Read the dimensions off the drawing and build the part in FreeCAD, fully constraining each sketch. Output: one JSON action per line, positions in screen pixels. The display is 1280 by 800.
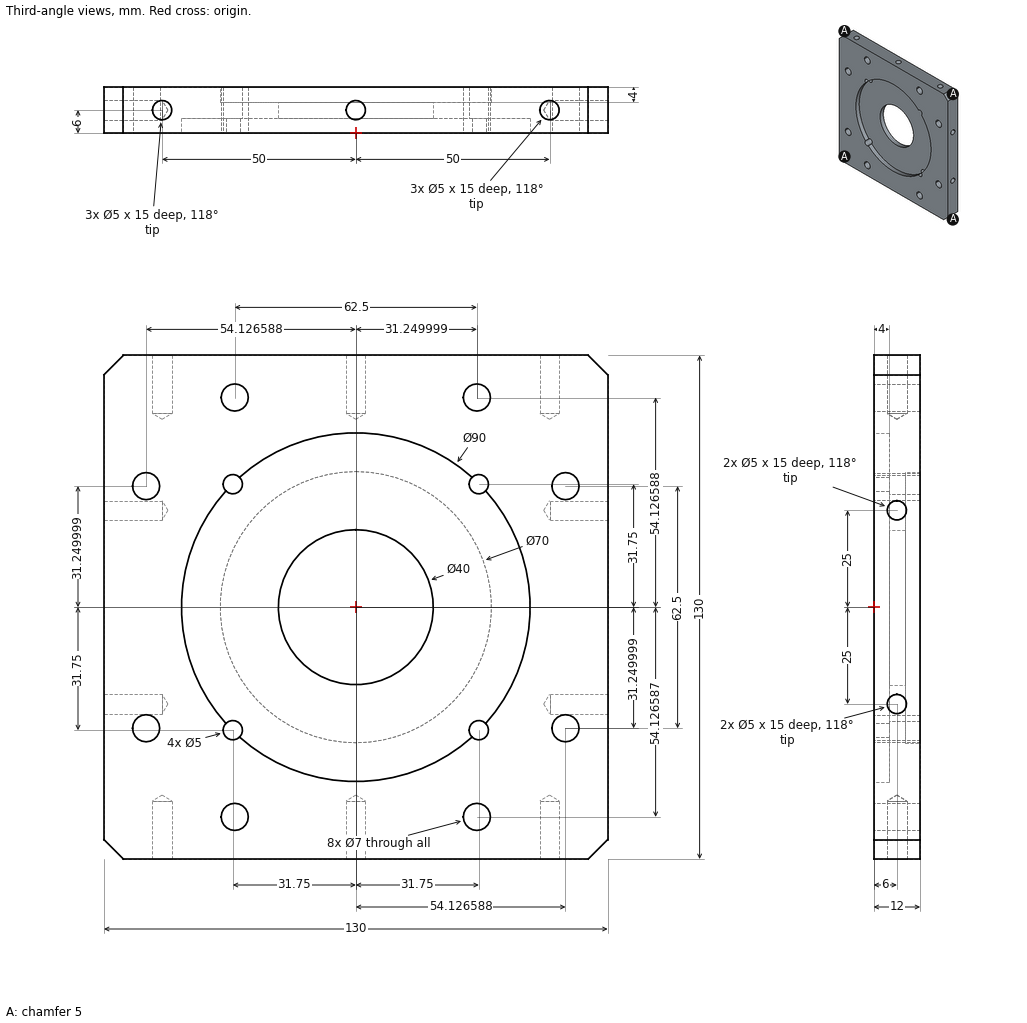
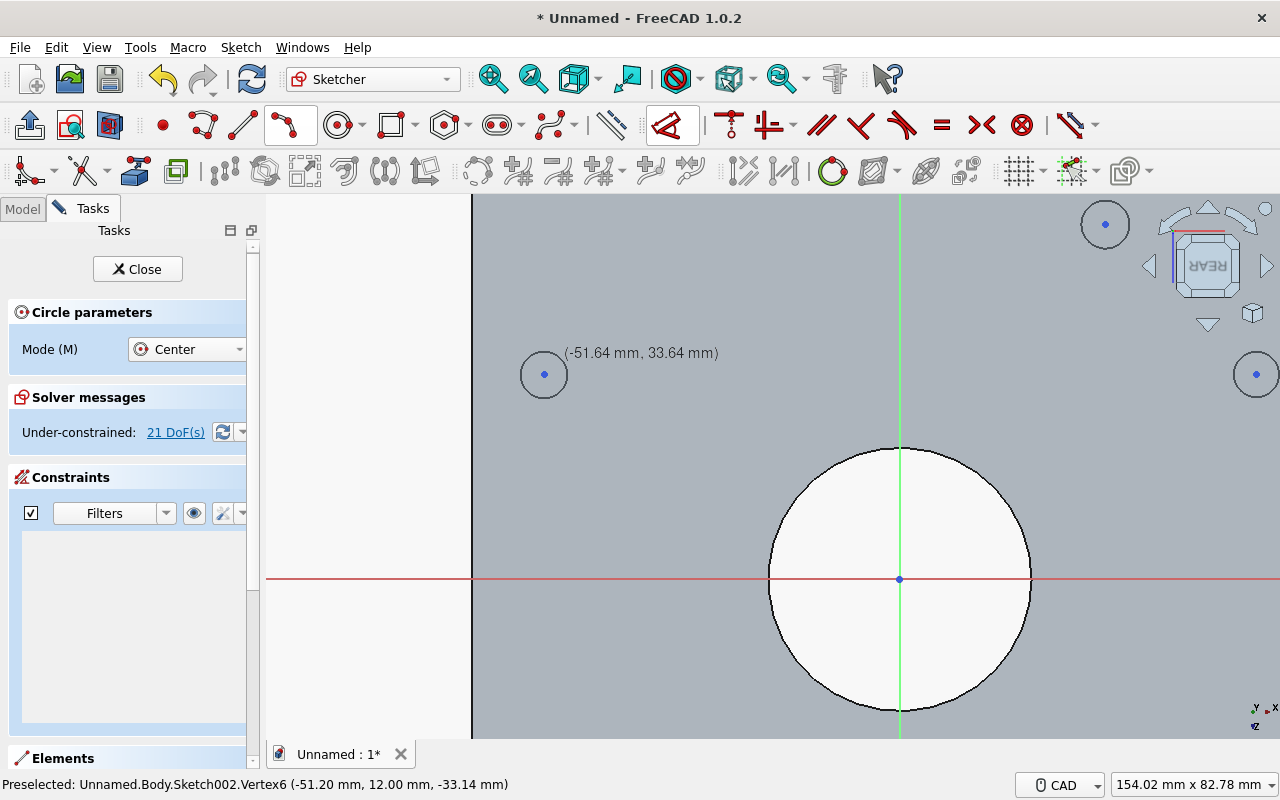
{"action": "left_click", "coordinate": [694, 223]}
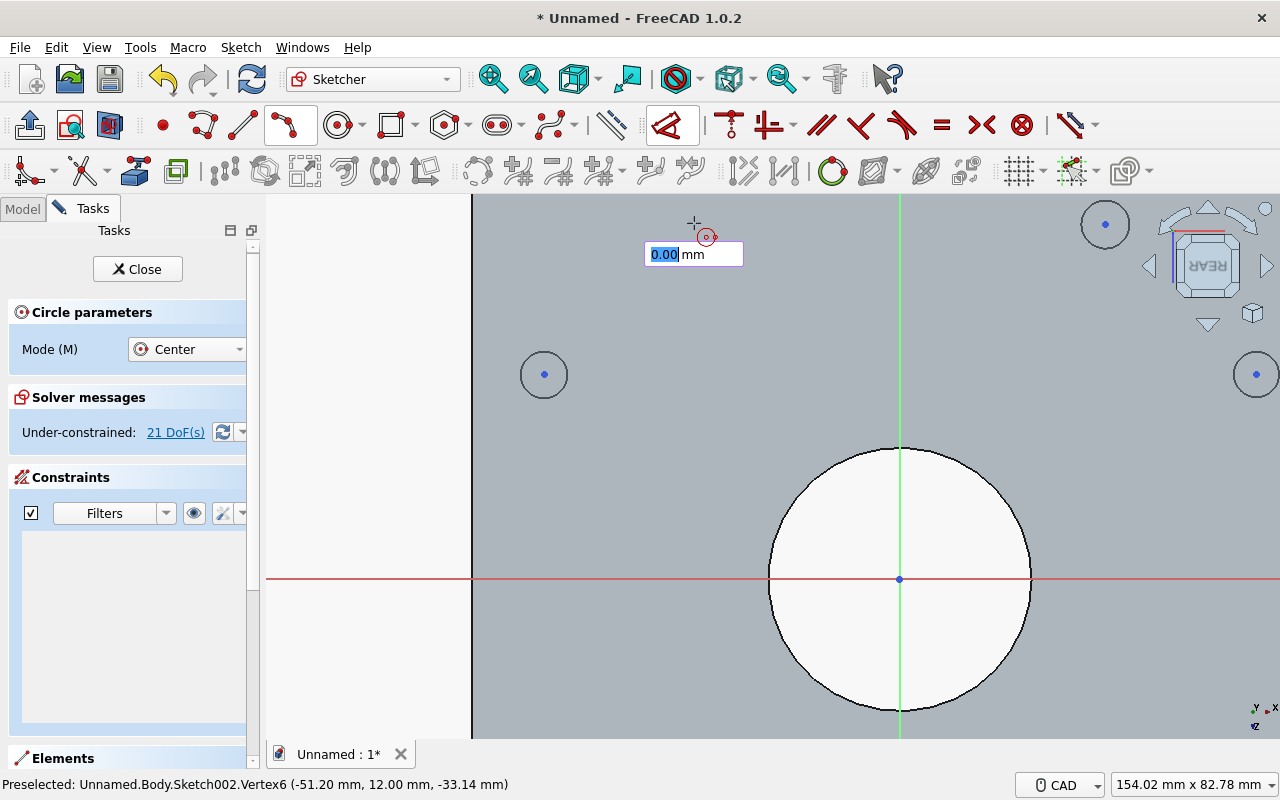
{"action": "scroll", "coordinate": [545, 374], "scroll_direction": "down", "scroll_amount": 4}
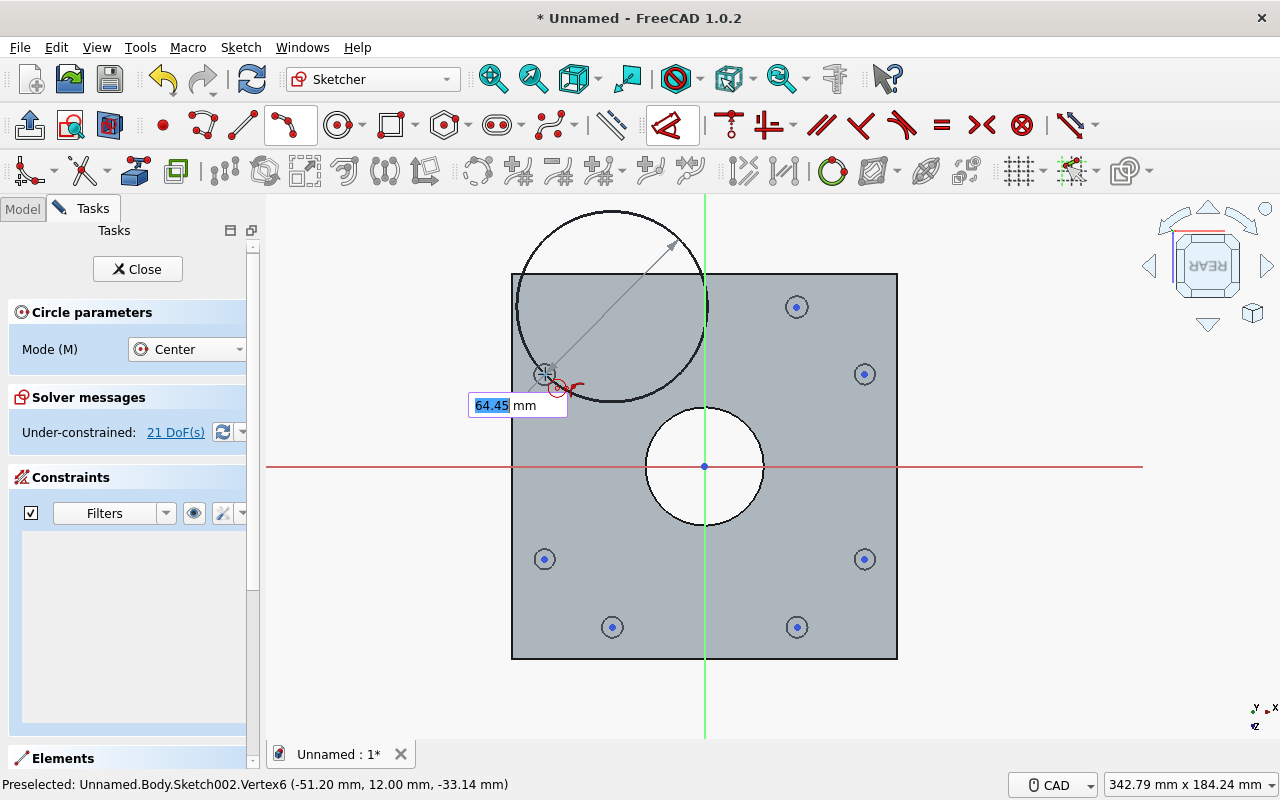
{"action": "scroll", "coordinate": [620, 299], "scroll_direction": "up", "scroll_amount": 3}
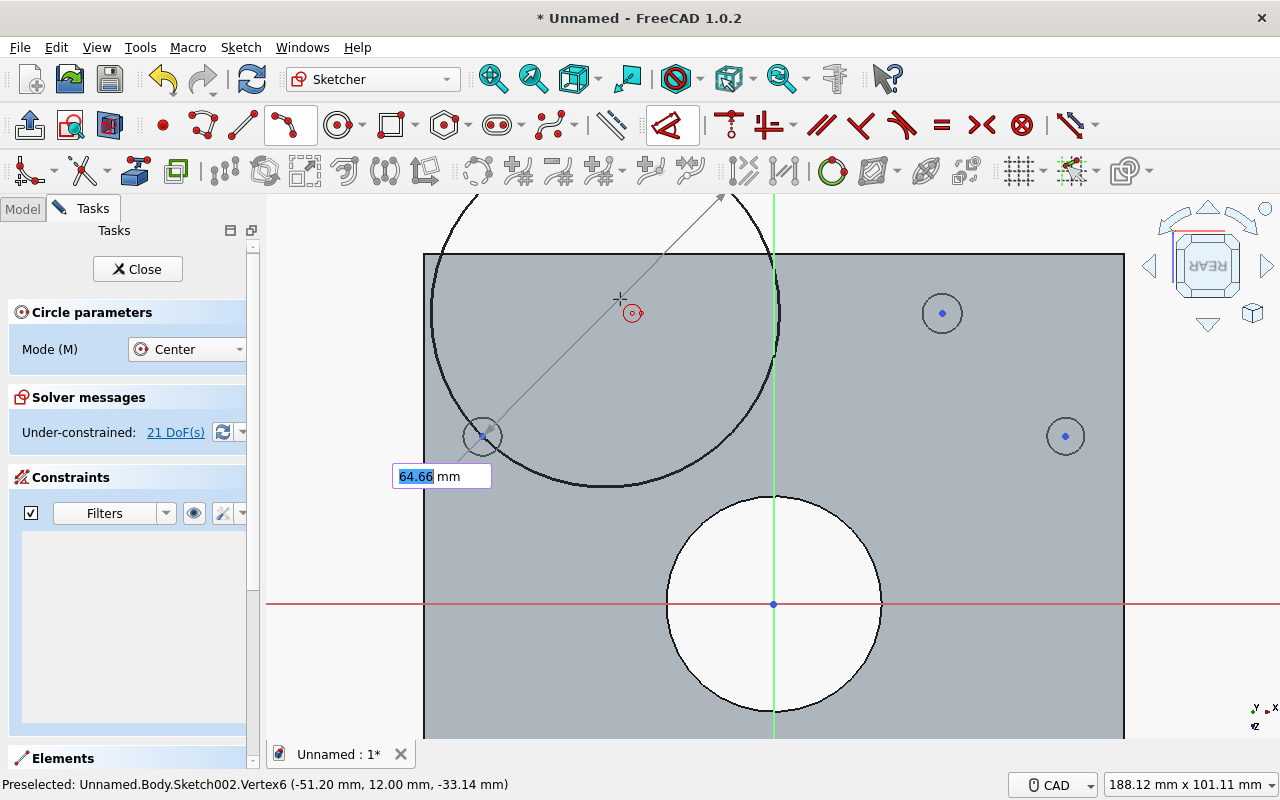
{"action": "left_click", "coordinate": [619, 299]}
{"action": "key", "text": "Escape"}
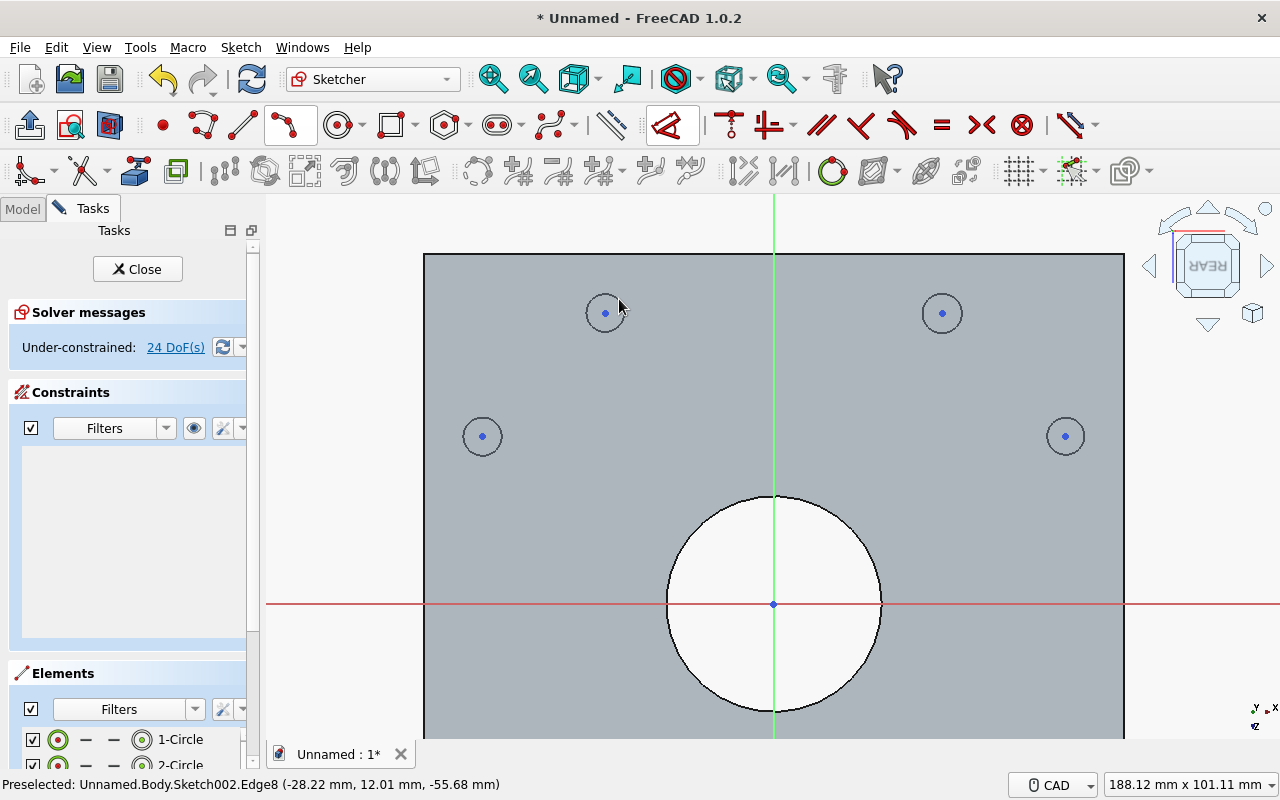
{"action": "left_click", "coordinate": [956, 299]}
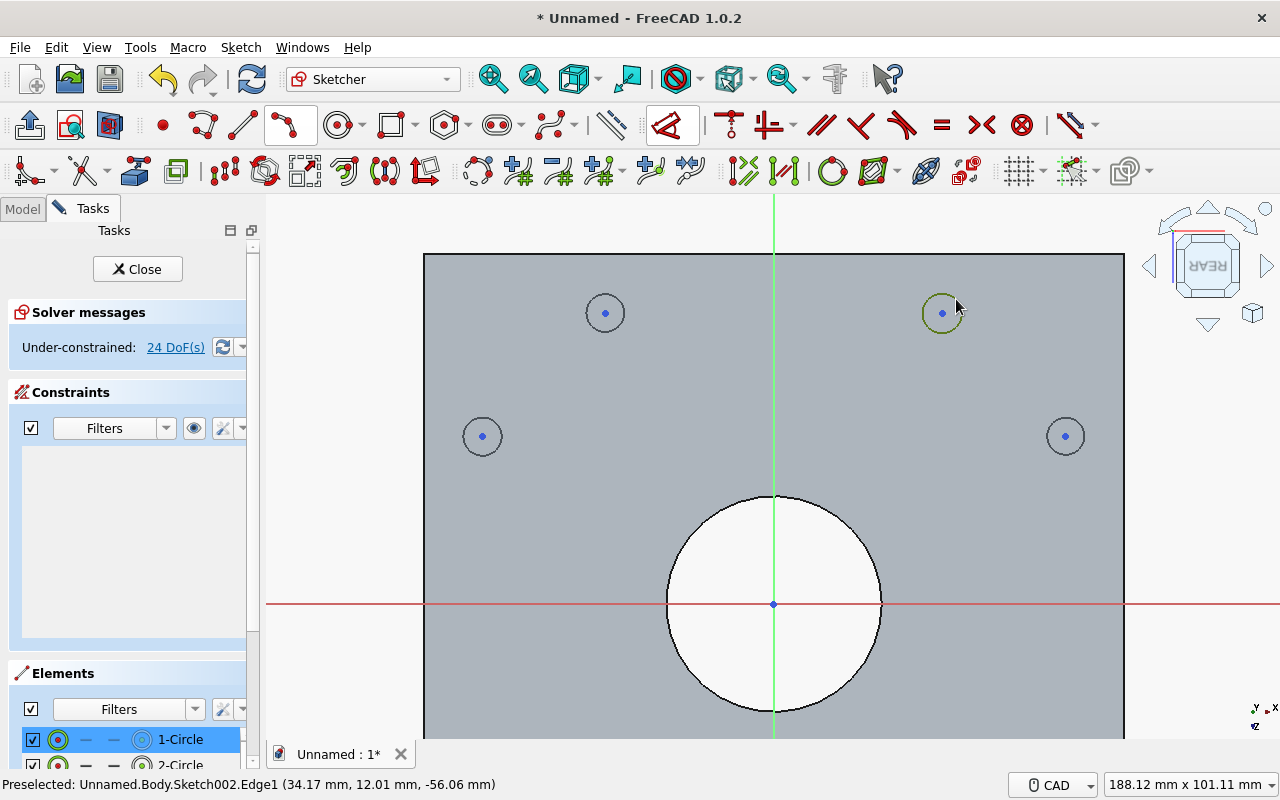
{"action": "left_click", "coordinate": [1079, 423]}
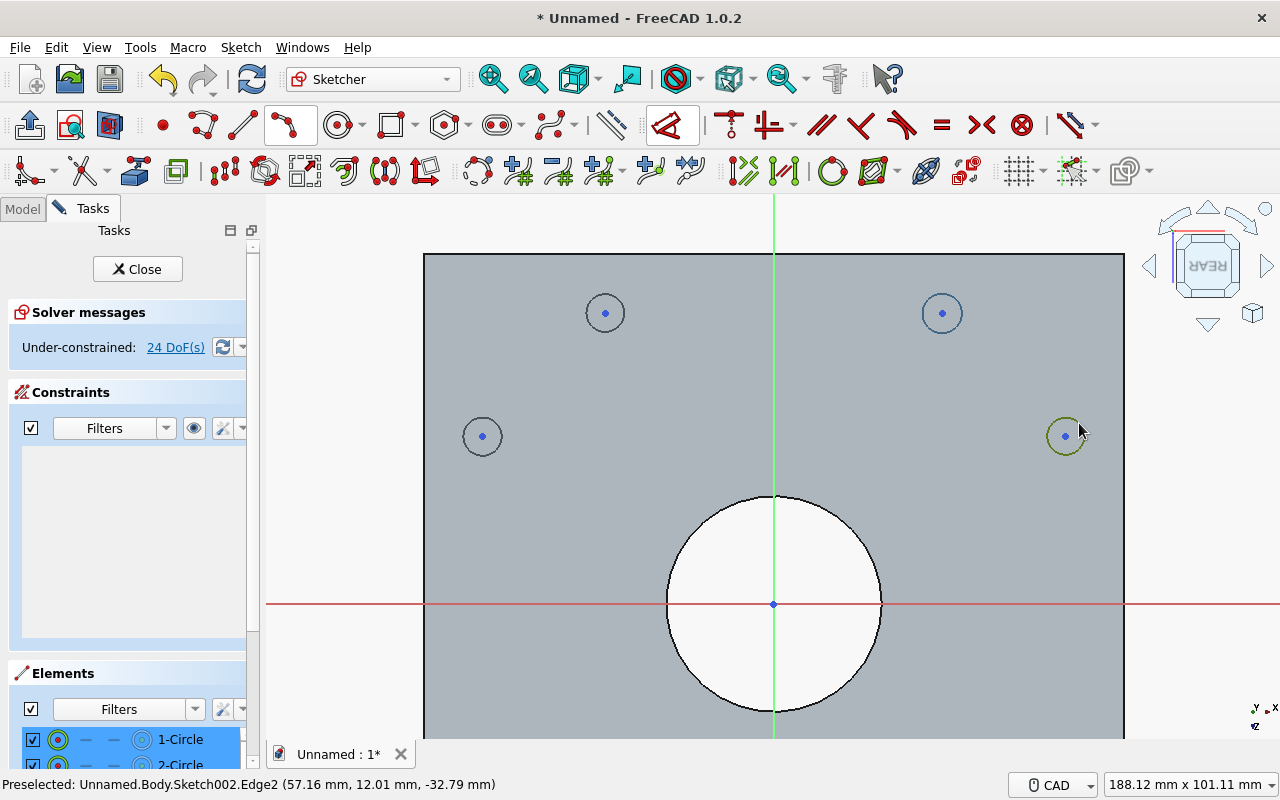
{"action": "scroll", "coordinate": [620, 299], "scroll_direction": "down", "scroll_amount": 3}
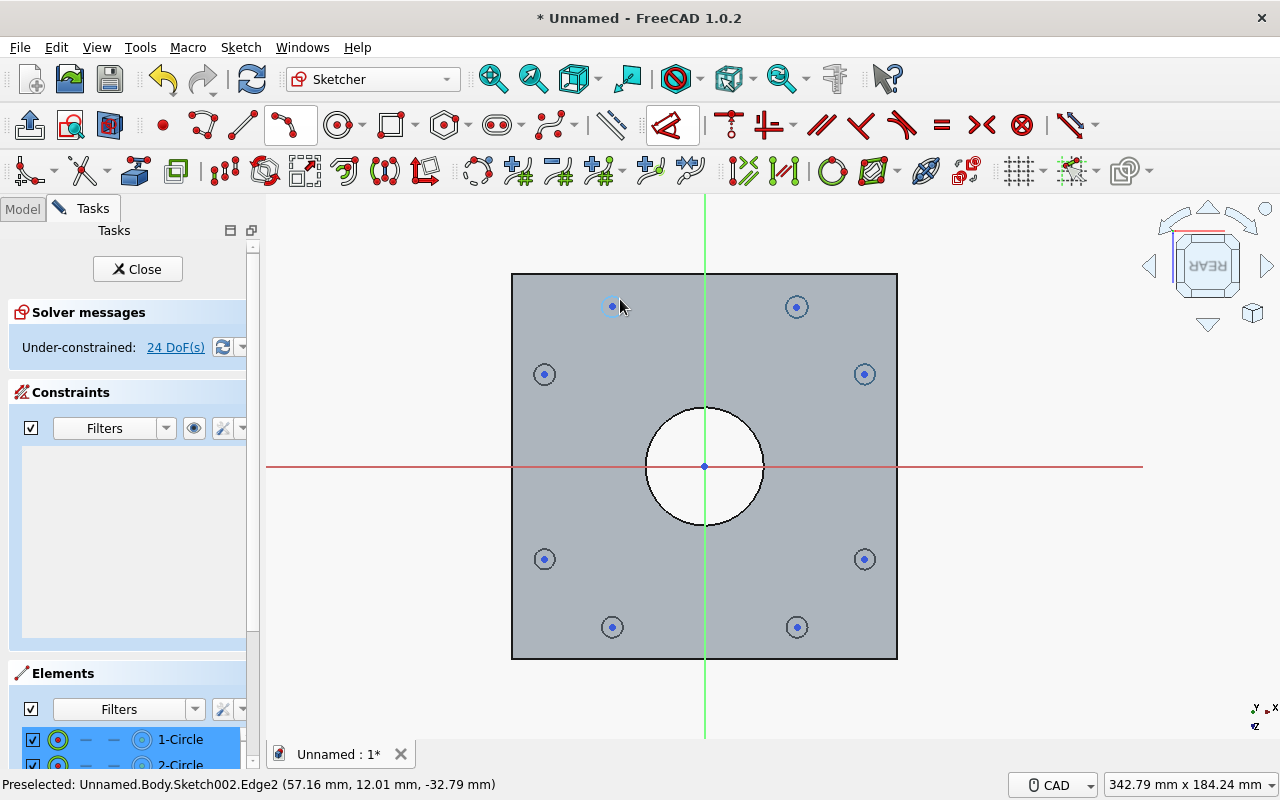
{"action": "scroll", "coordinate": [872, 552], "scroll_direction": "up", "scroll_amount": 2}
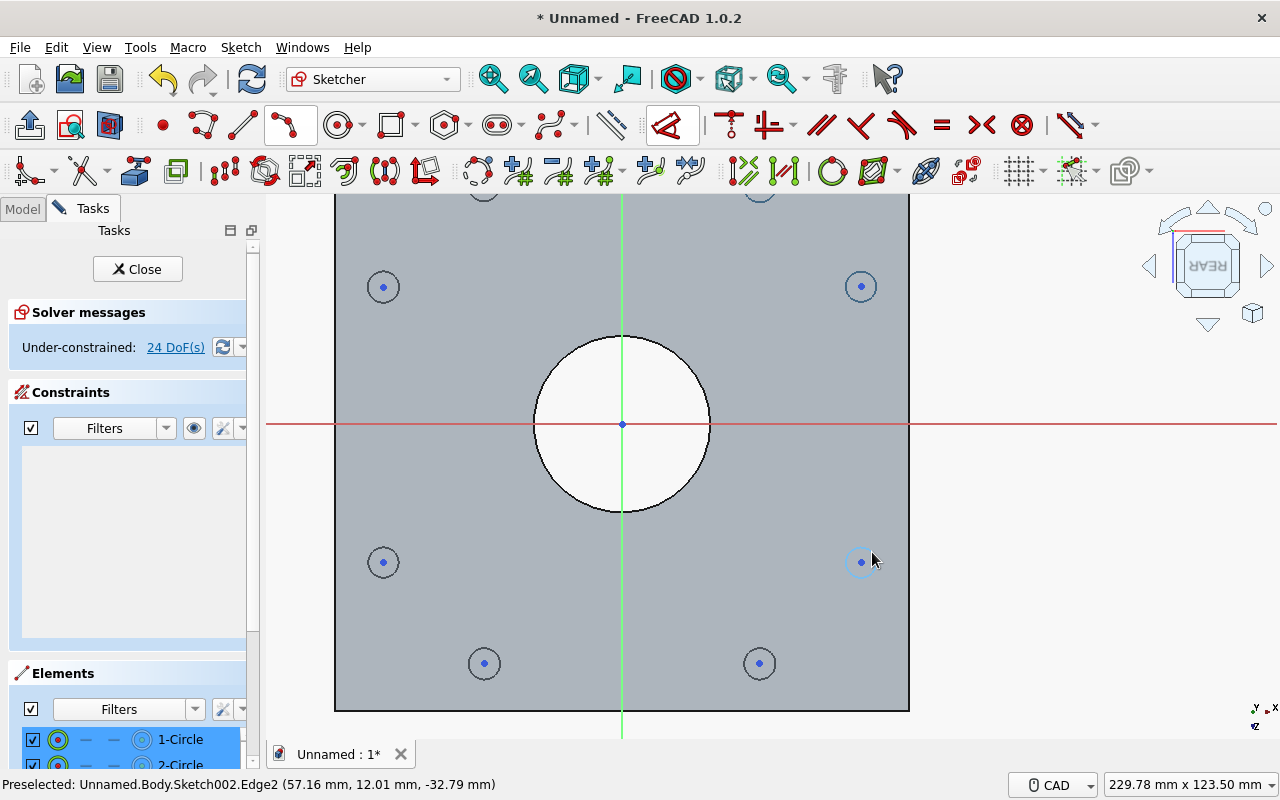
{"action": "left_click", "coordinate": [872, 552]}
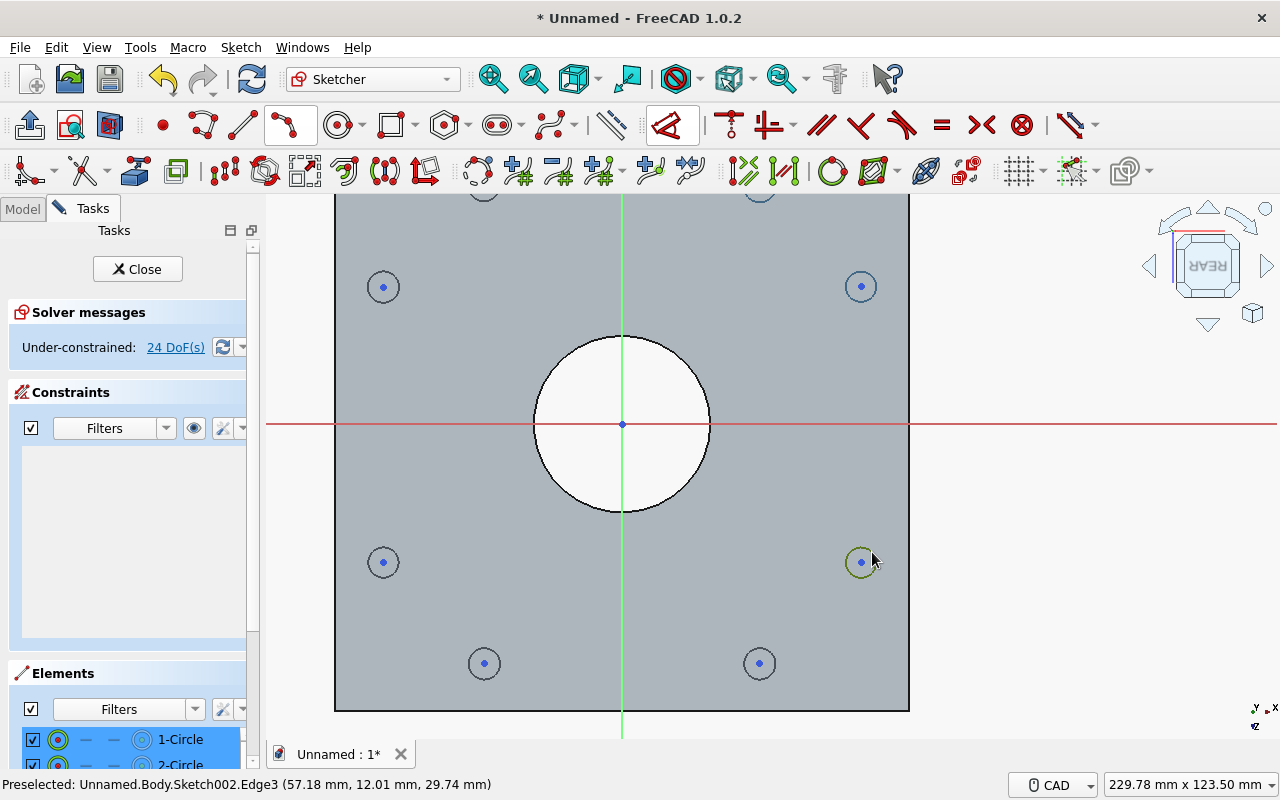
{"action": "left_click", "coordinate": [771, 653]}